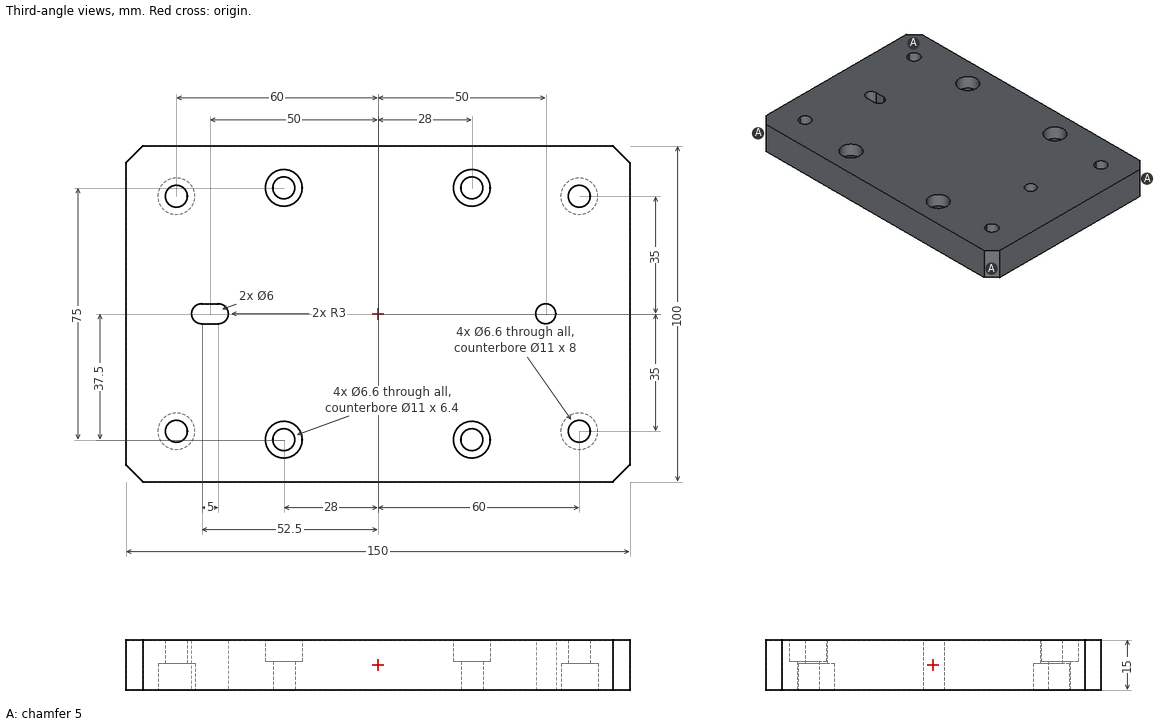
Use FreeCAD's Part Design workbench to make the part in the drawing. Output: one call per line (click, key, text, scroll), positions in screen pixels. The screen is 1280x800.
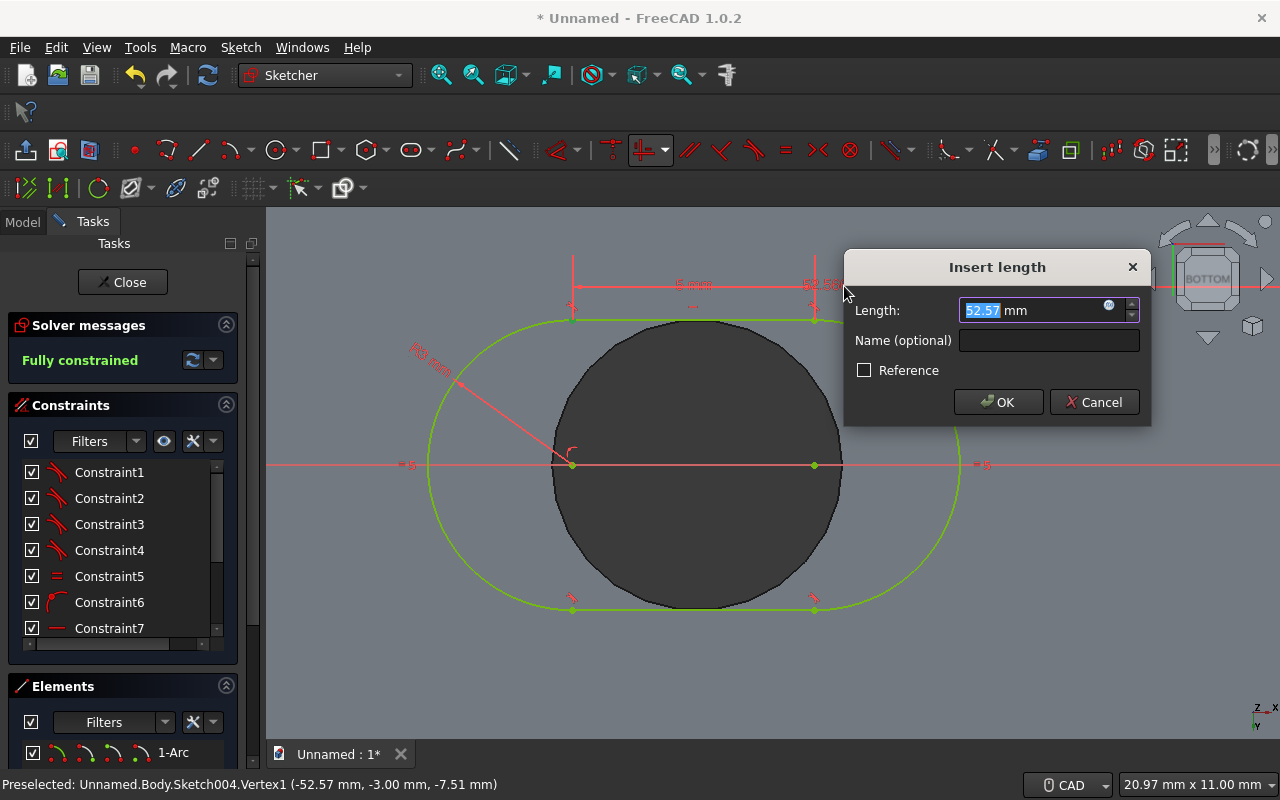
text(52.5)
key(Return)
key(Escape)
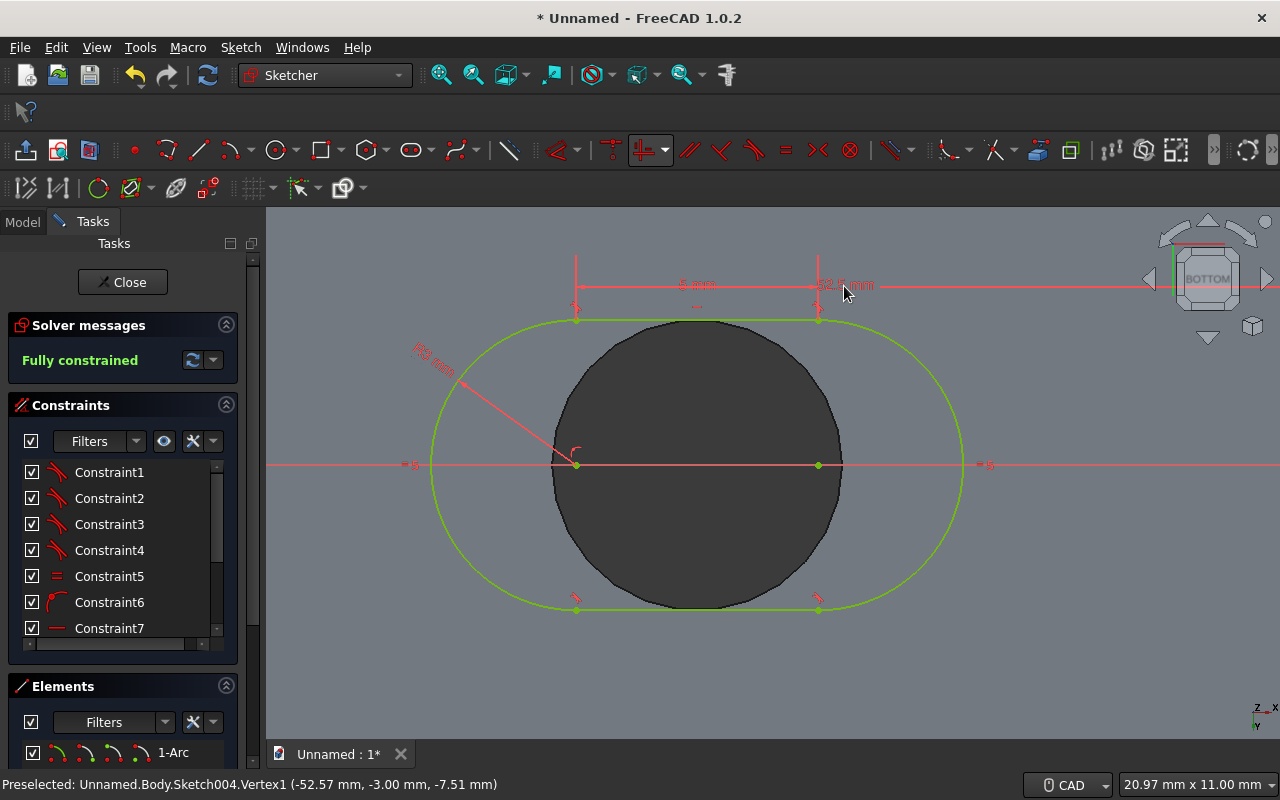
click(123, 282)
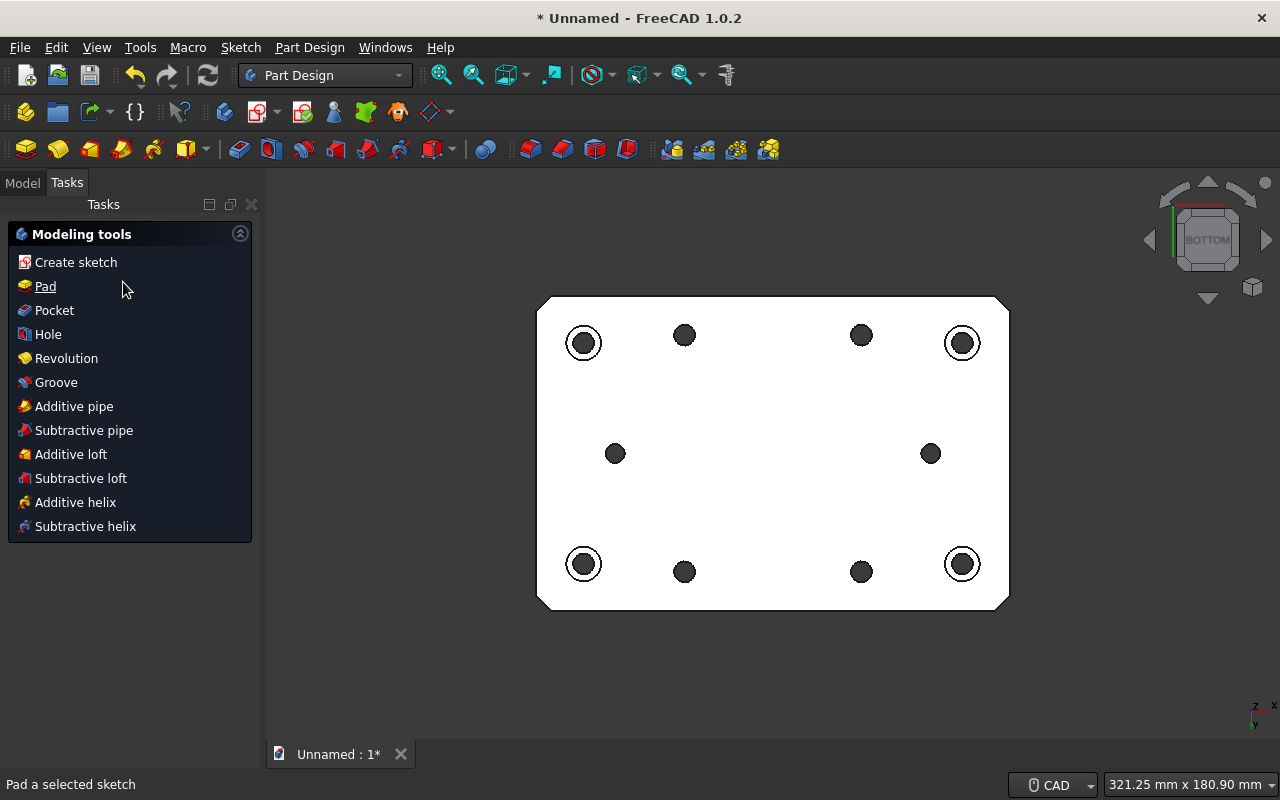
click(240, 150)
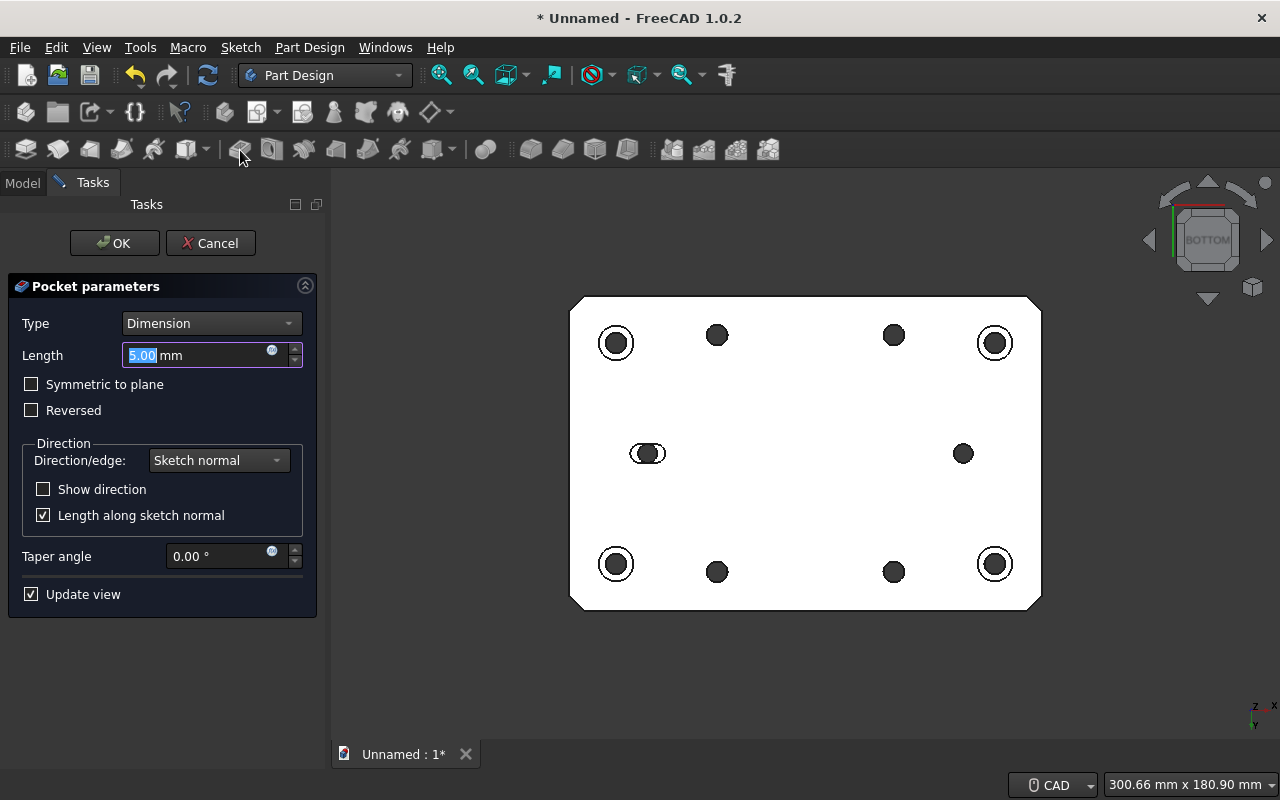
click(212, 324)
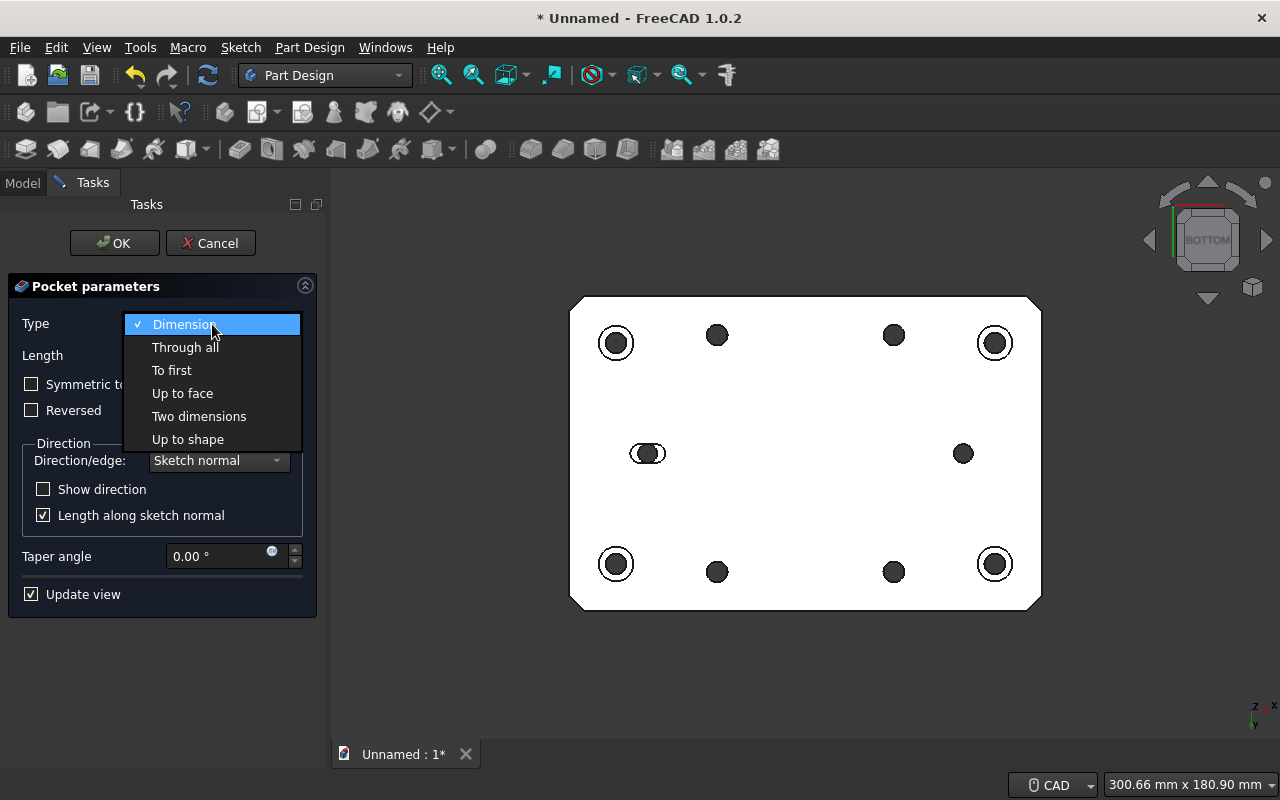
click(212, 348)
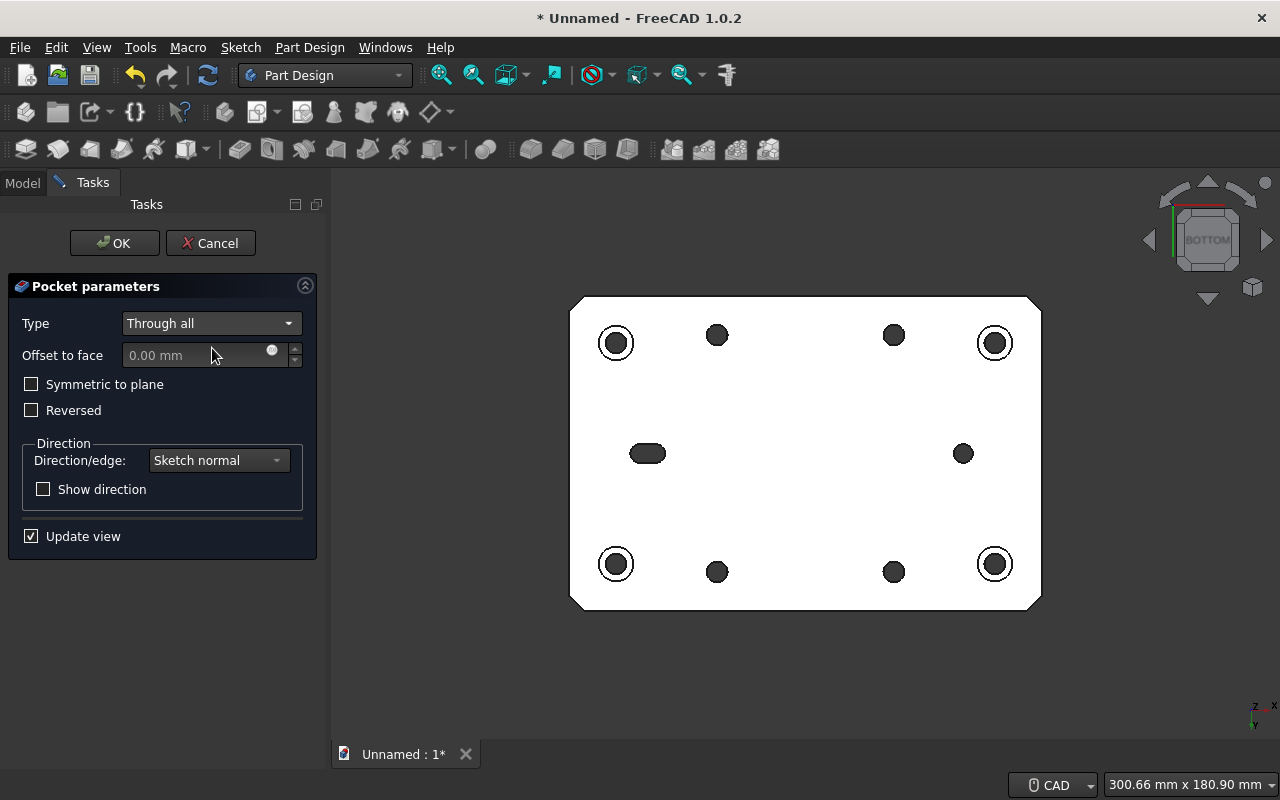
click(115, 243)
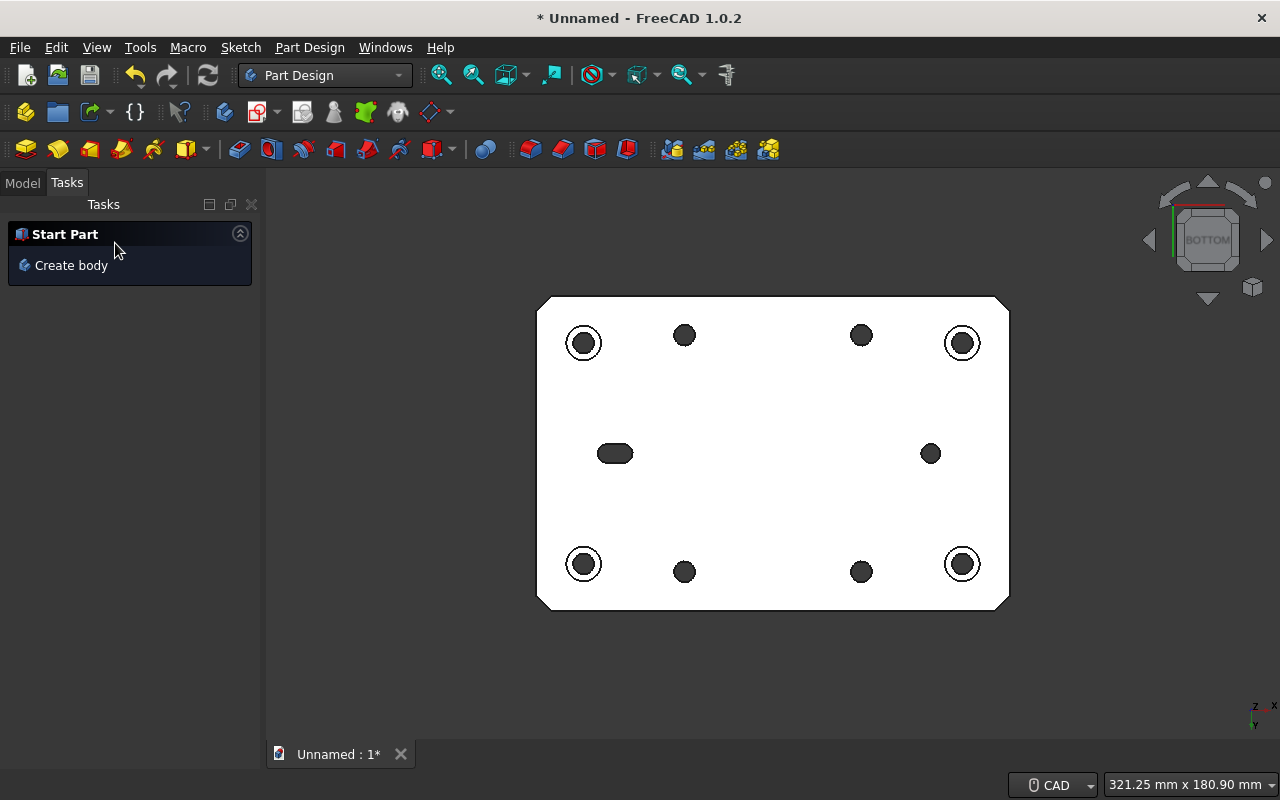
key(0)